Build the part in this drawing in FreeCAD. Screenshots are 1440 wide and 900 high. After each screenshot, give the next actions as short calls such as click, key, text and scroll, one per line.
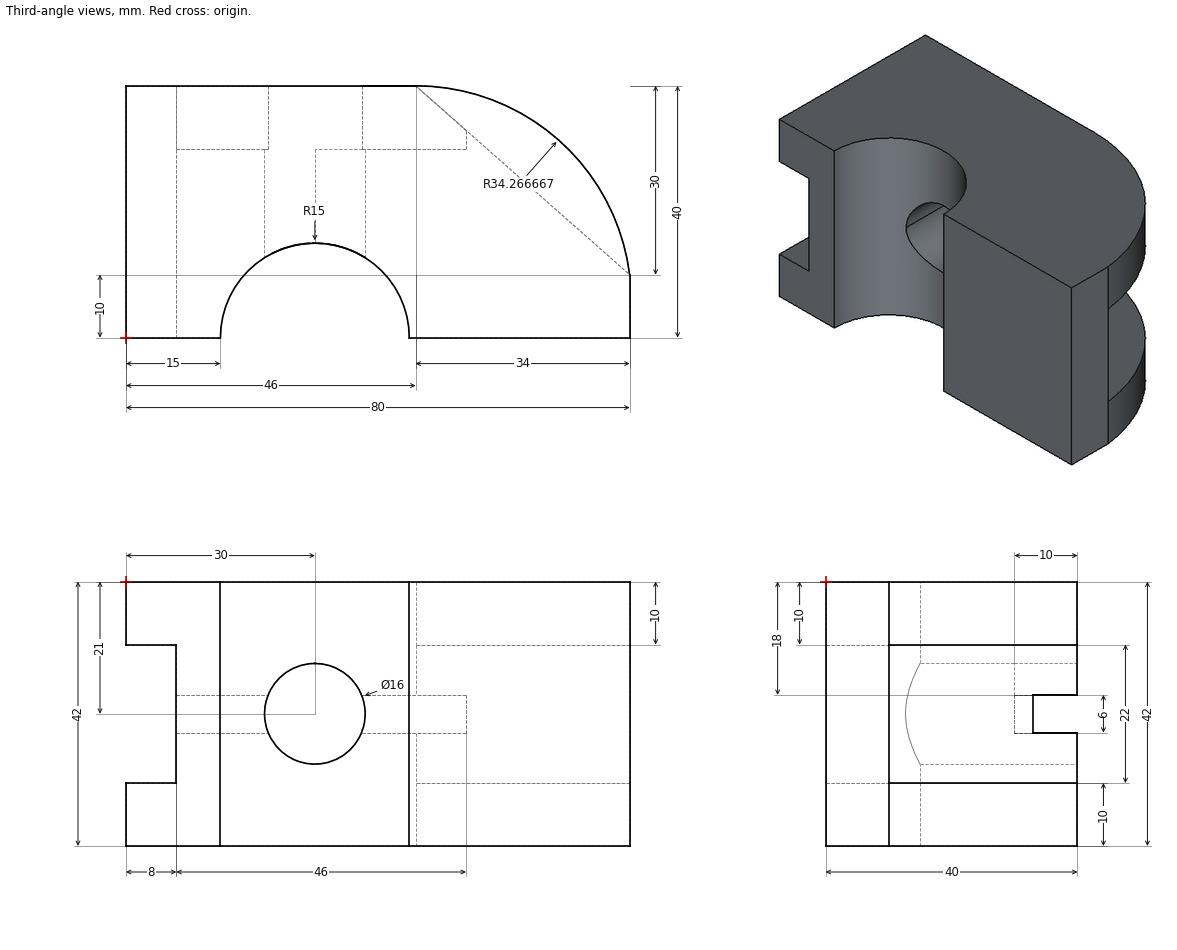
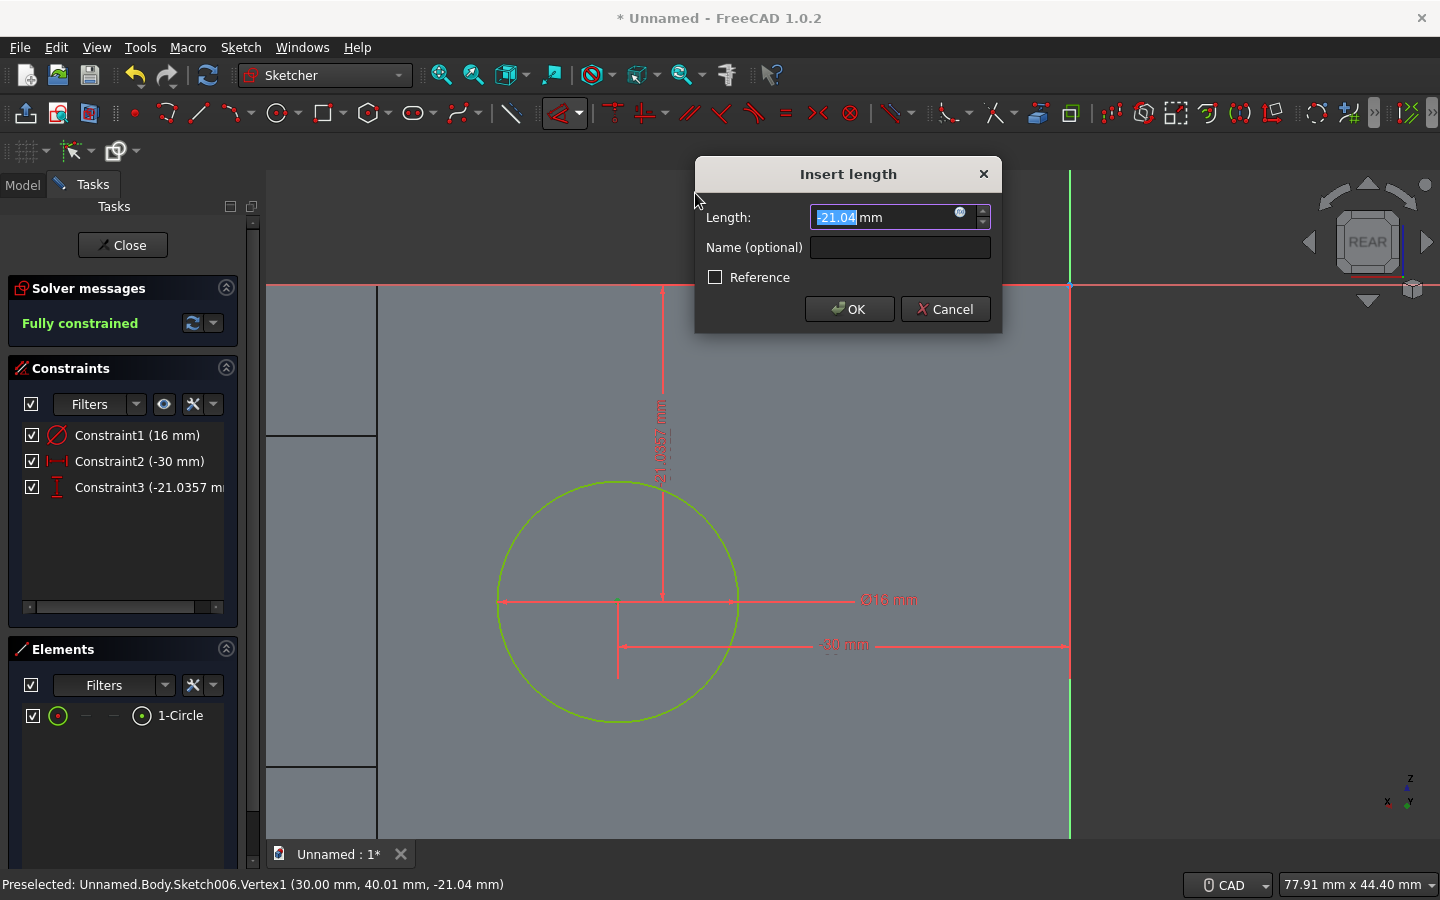
text(-21)
key(Return)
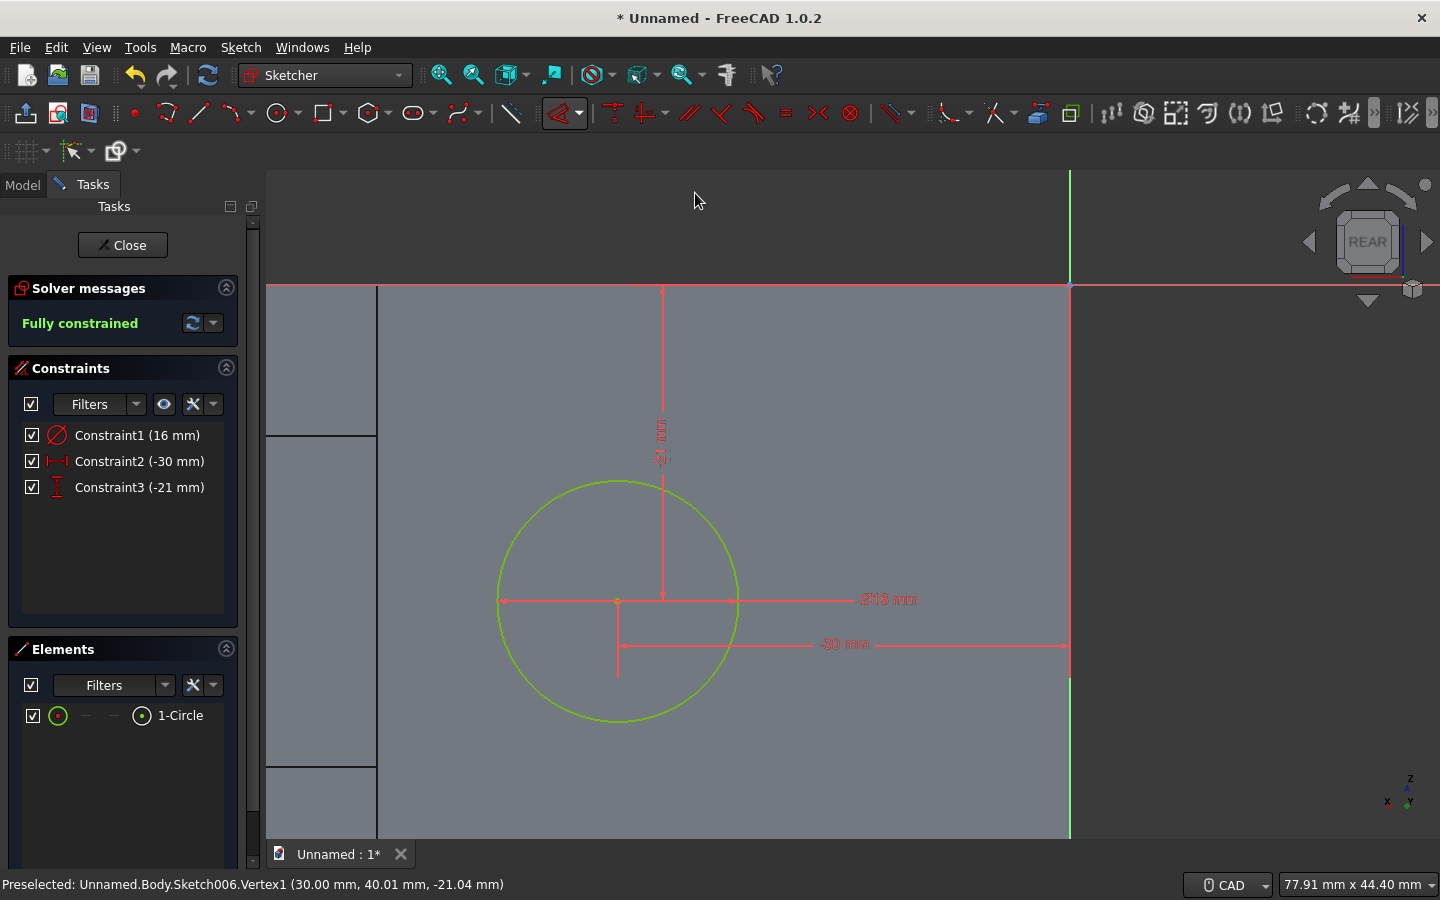
click(123, 245)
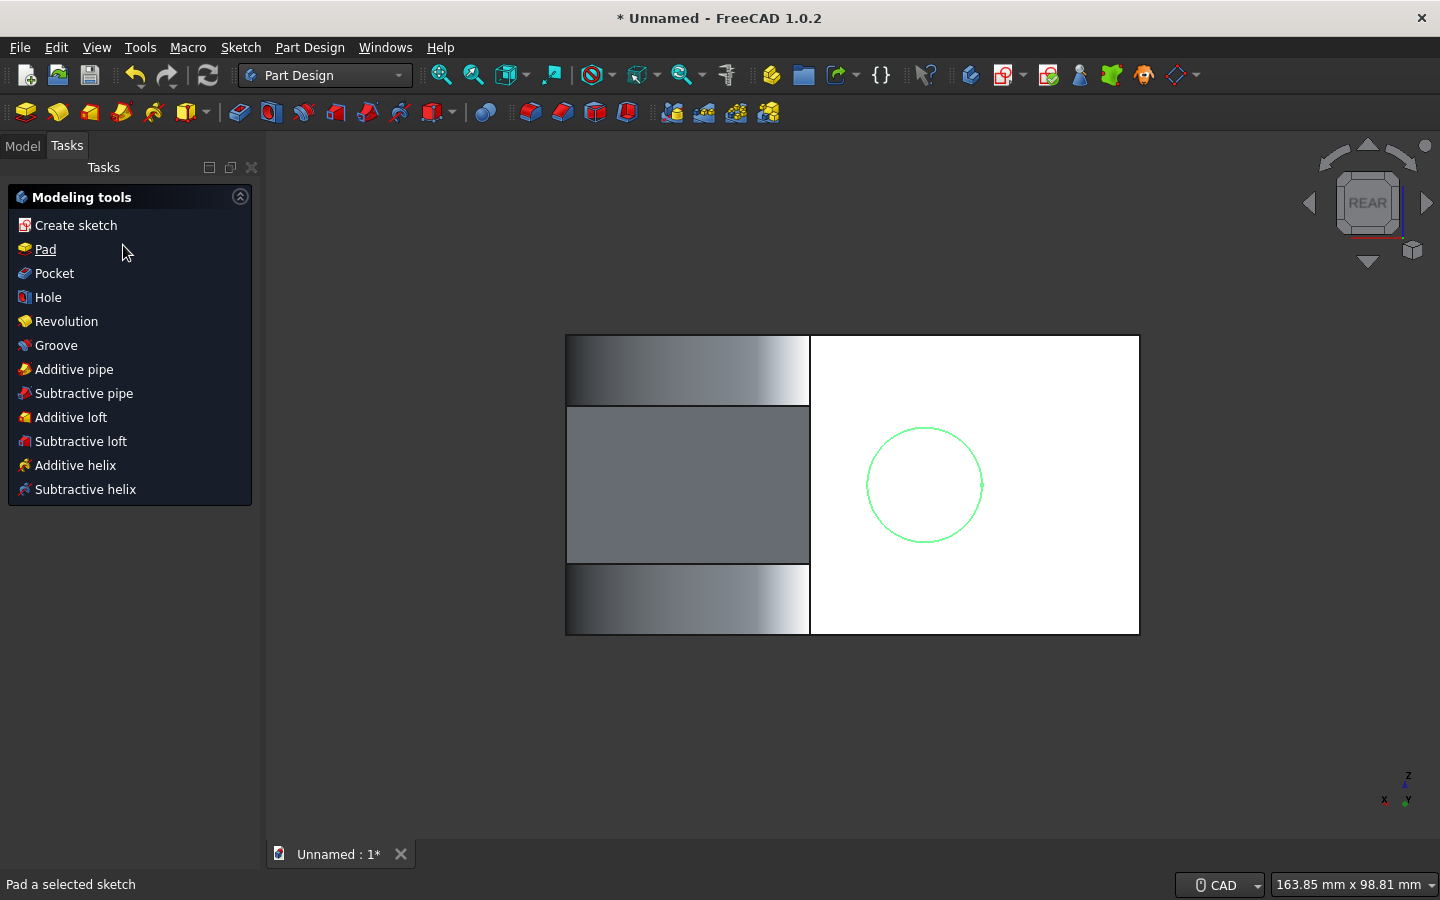
click(240, 112)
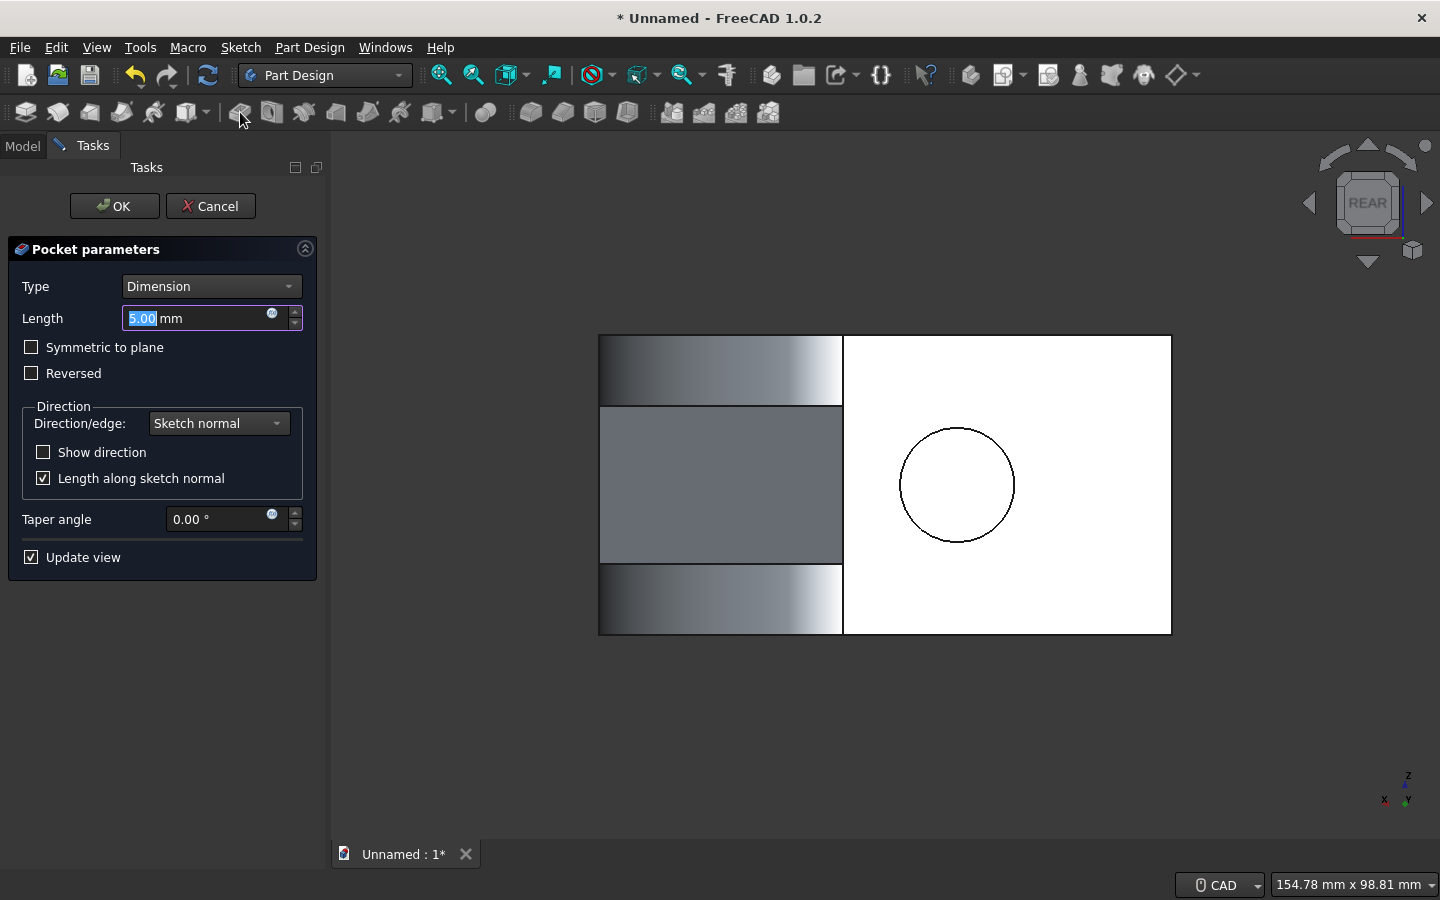
text(10)
key(Tab)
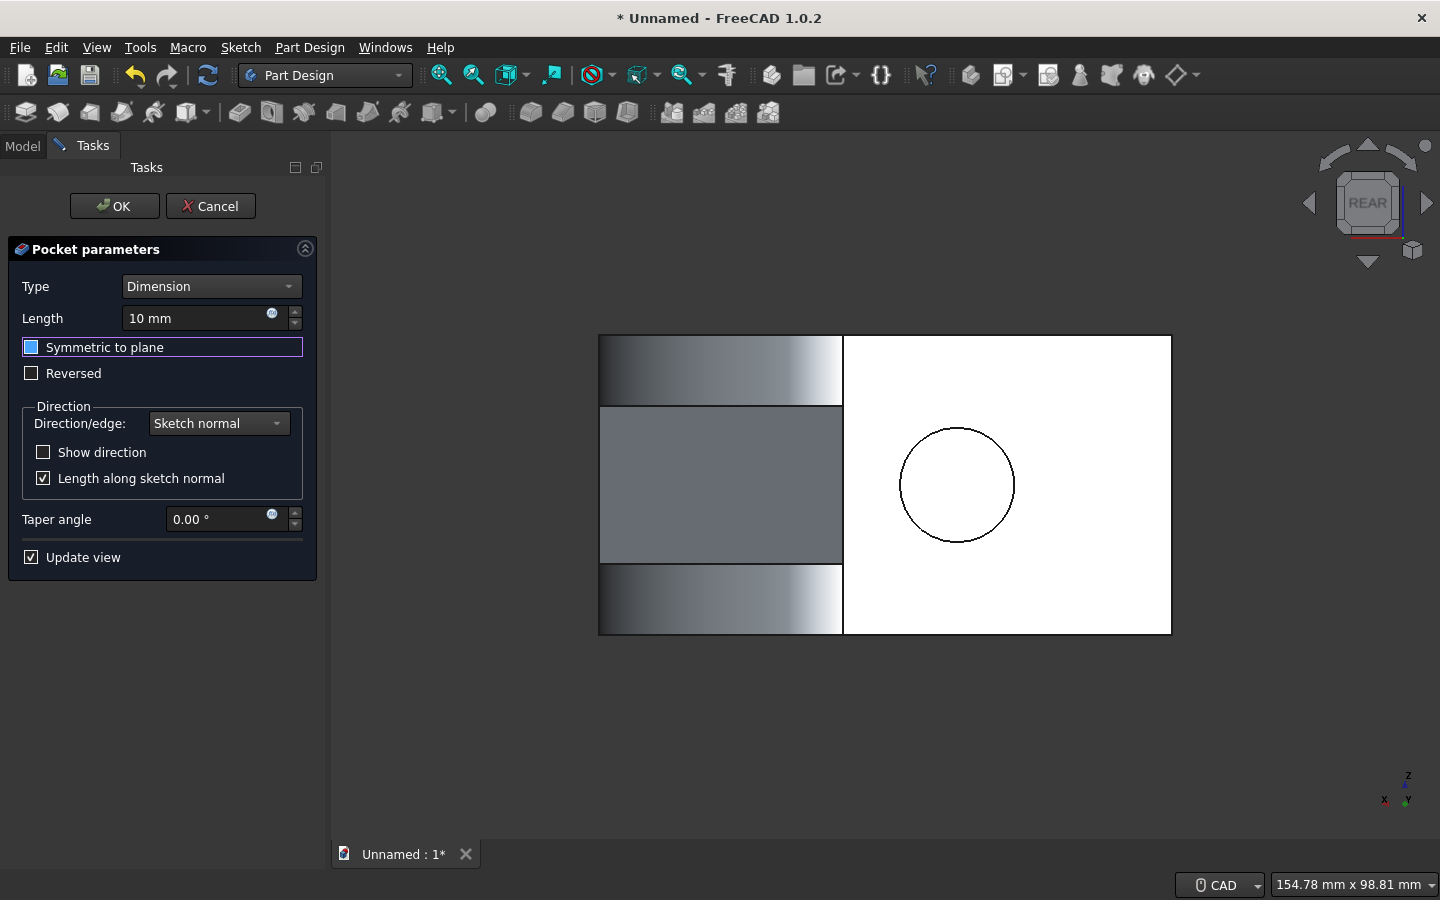
click(115, 206)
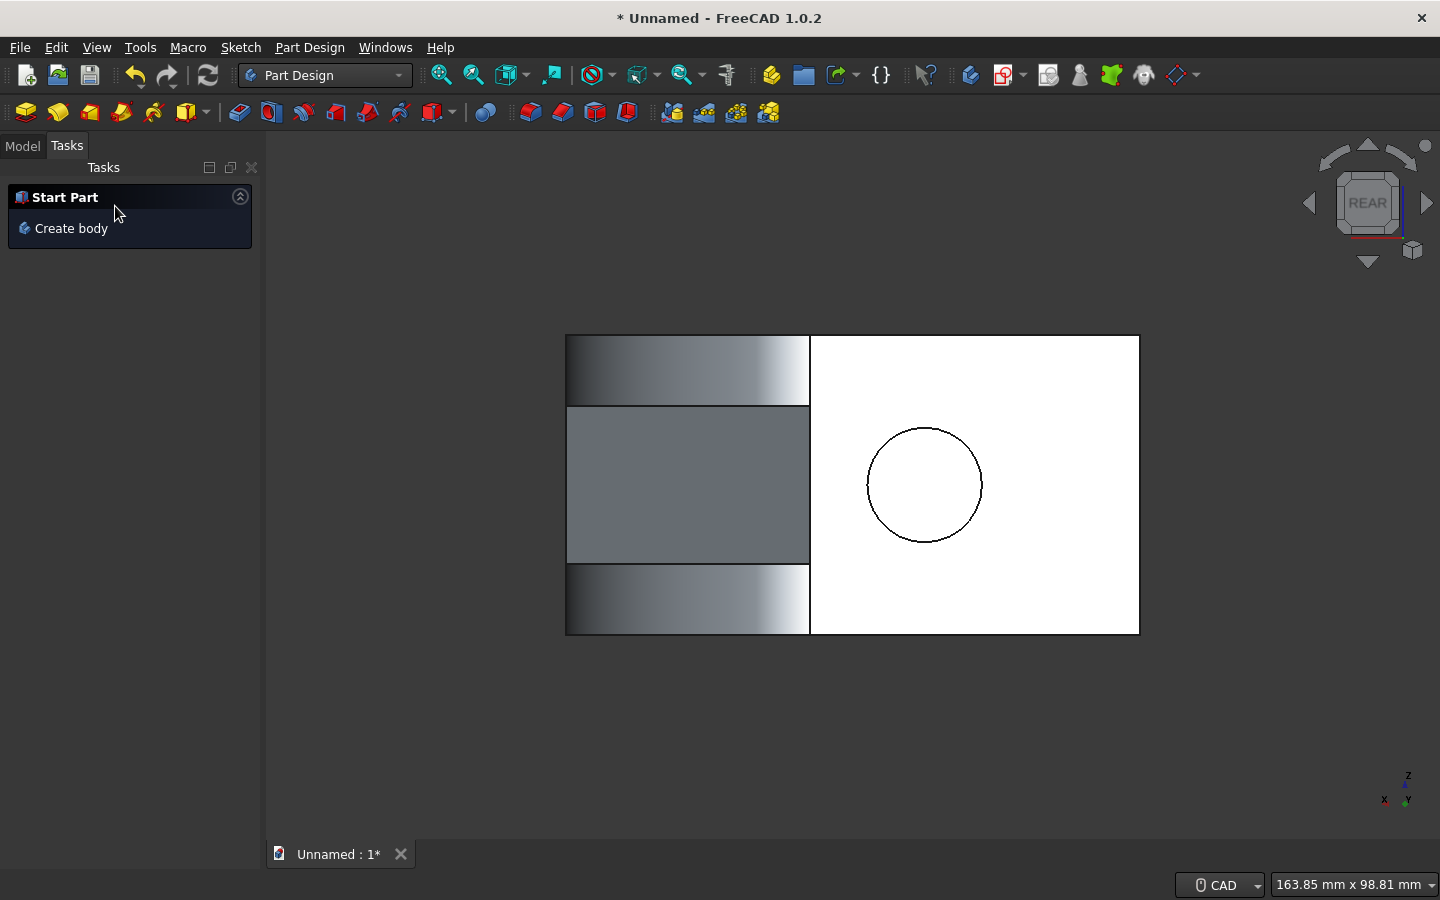
click(1004, 76)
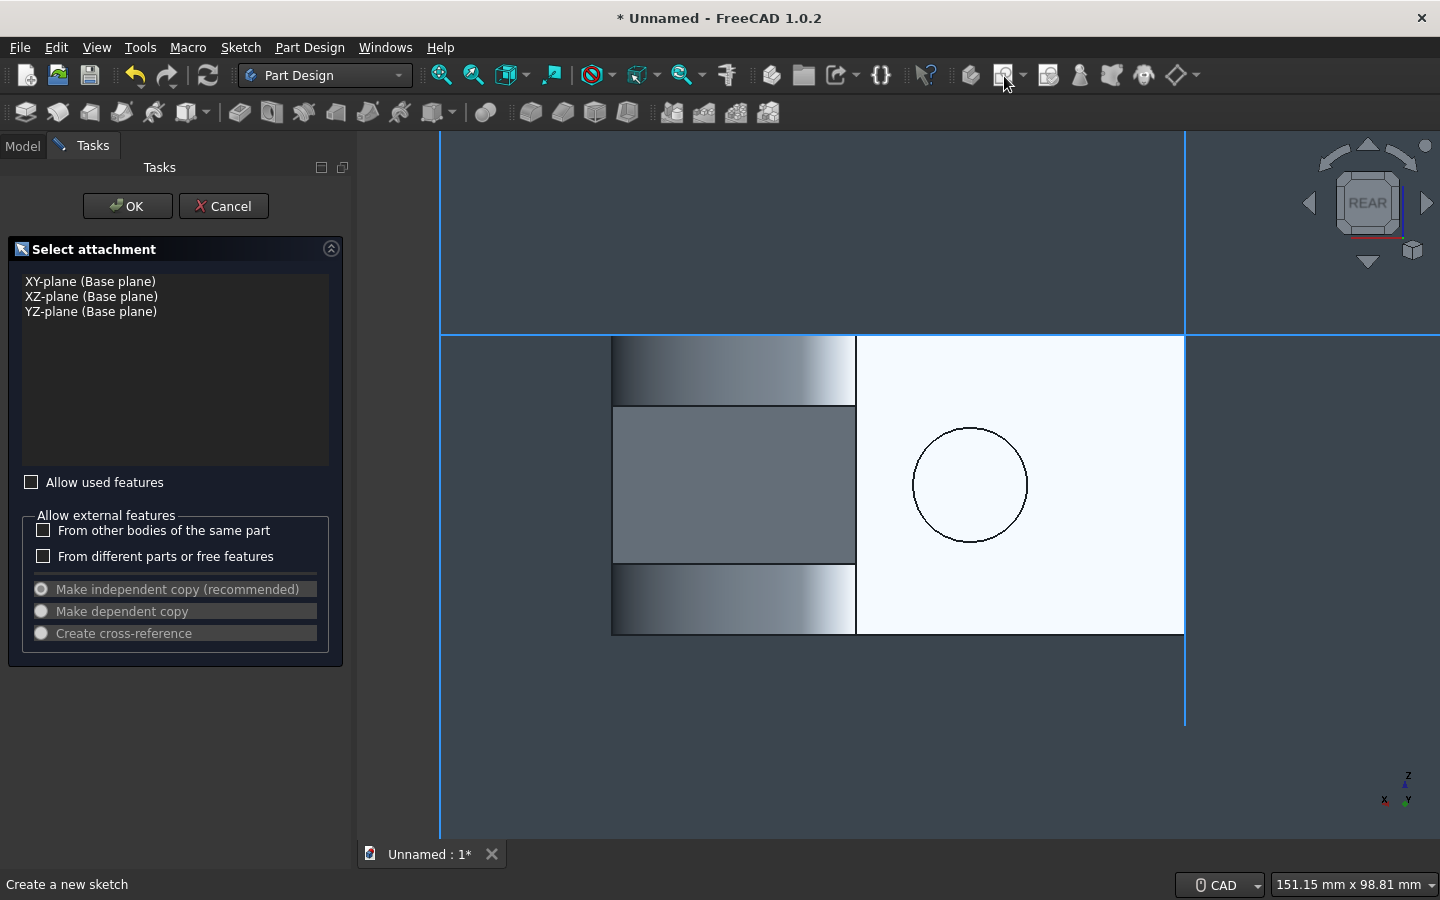
click(82, 312)